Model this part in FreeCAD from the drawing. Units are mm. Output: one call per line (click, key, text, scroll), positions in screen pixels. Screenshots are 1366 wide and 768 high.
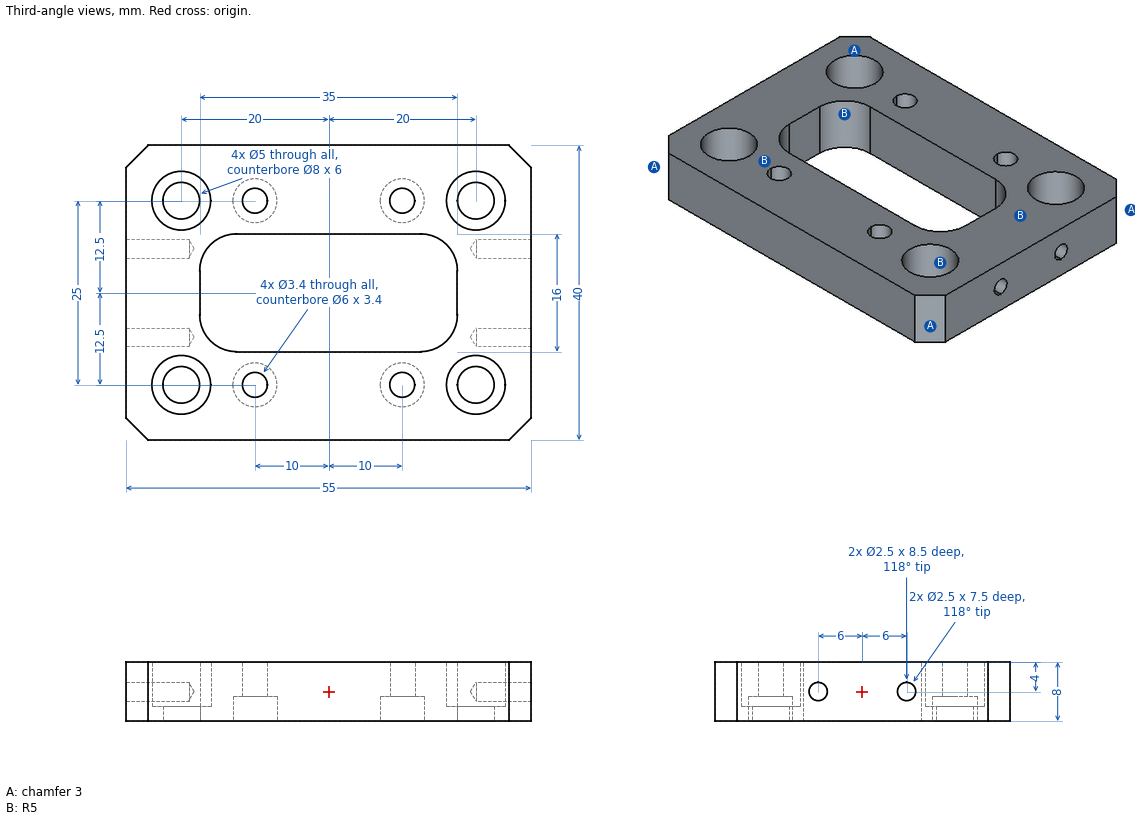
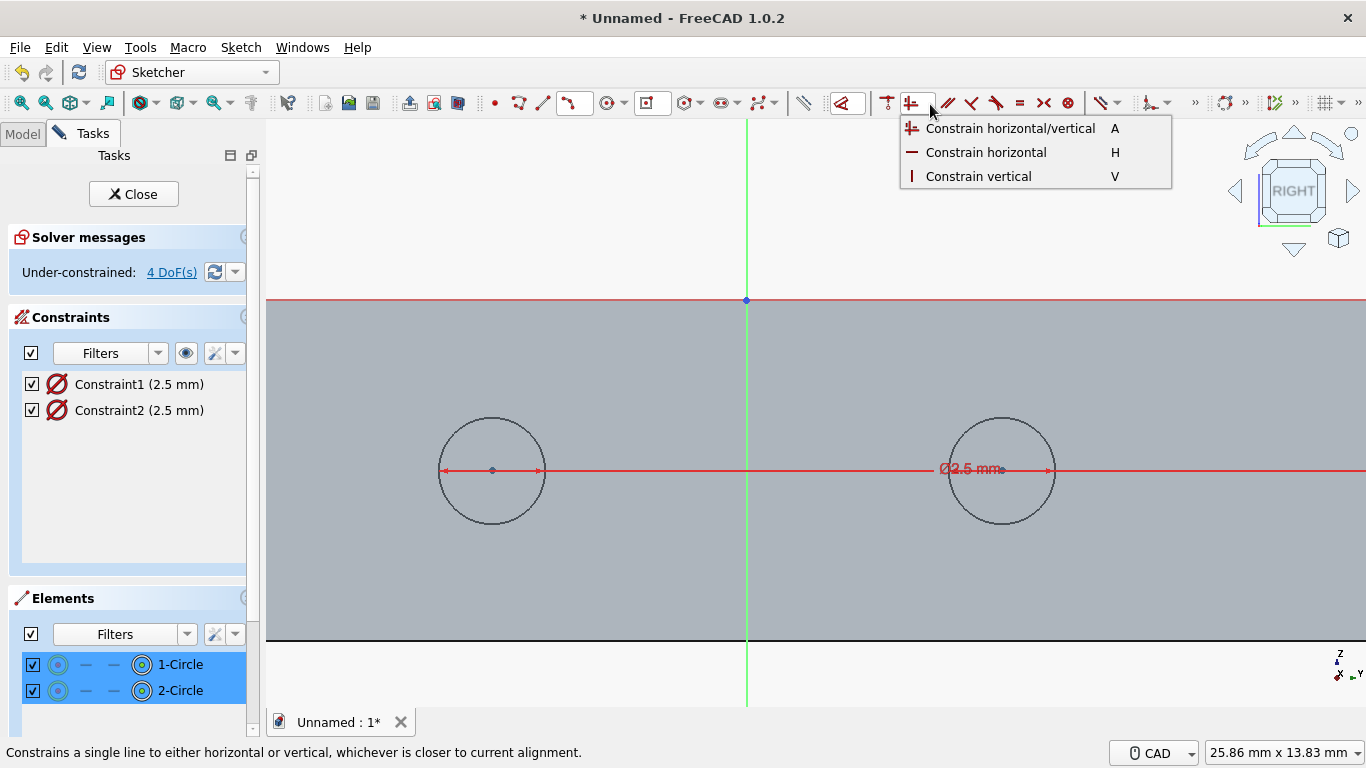
click(1036, 152)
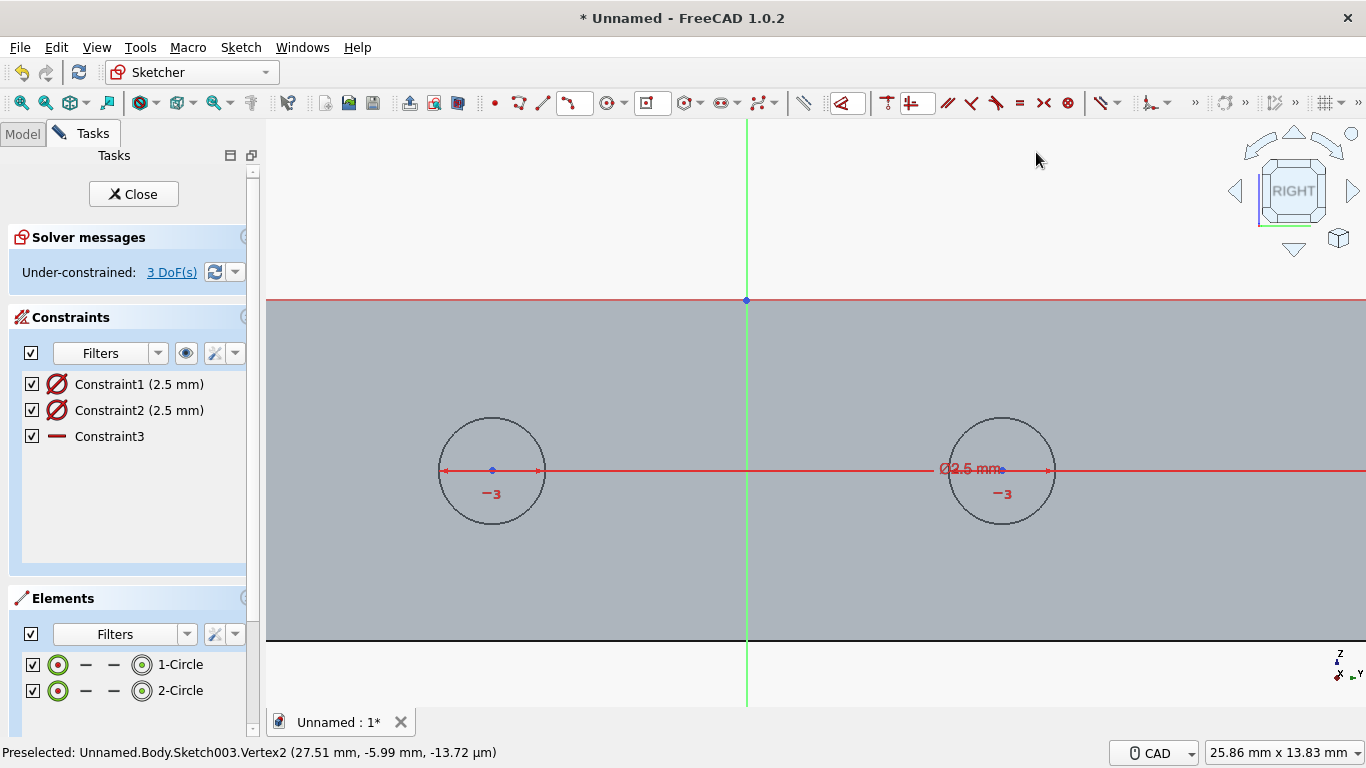
click(1002, 471)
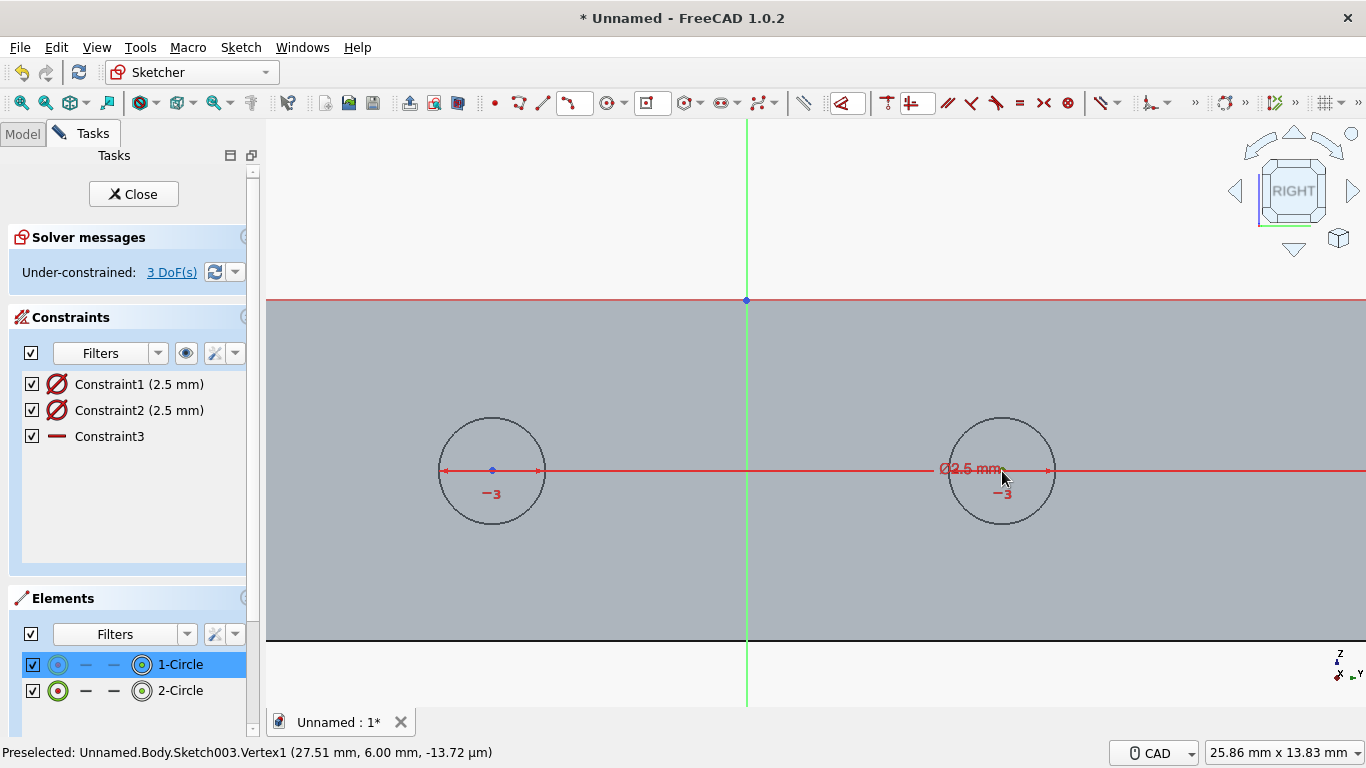
click(860, 104)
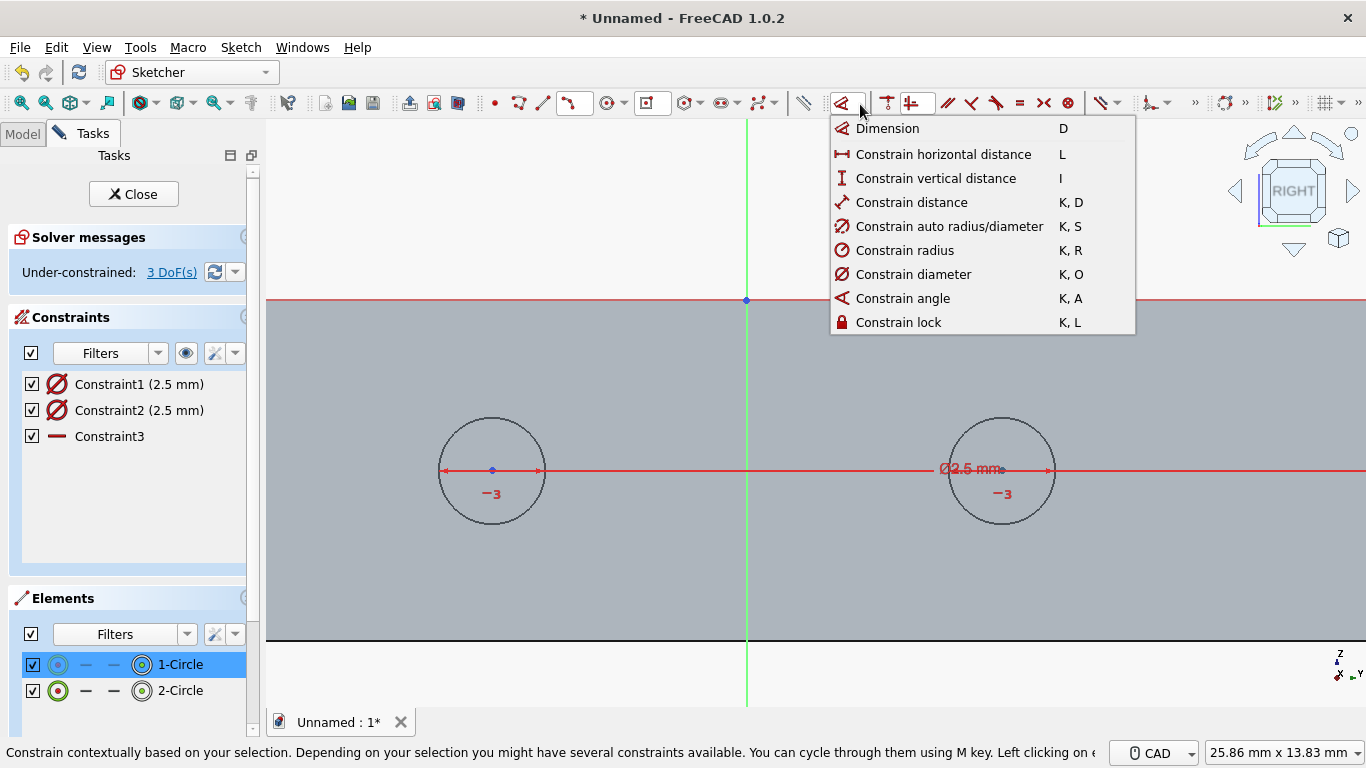
click(983, 154)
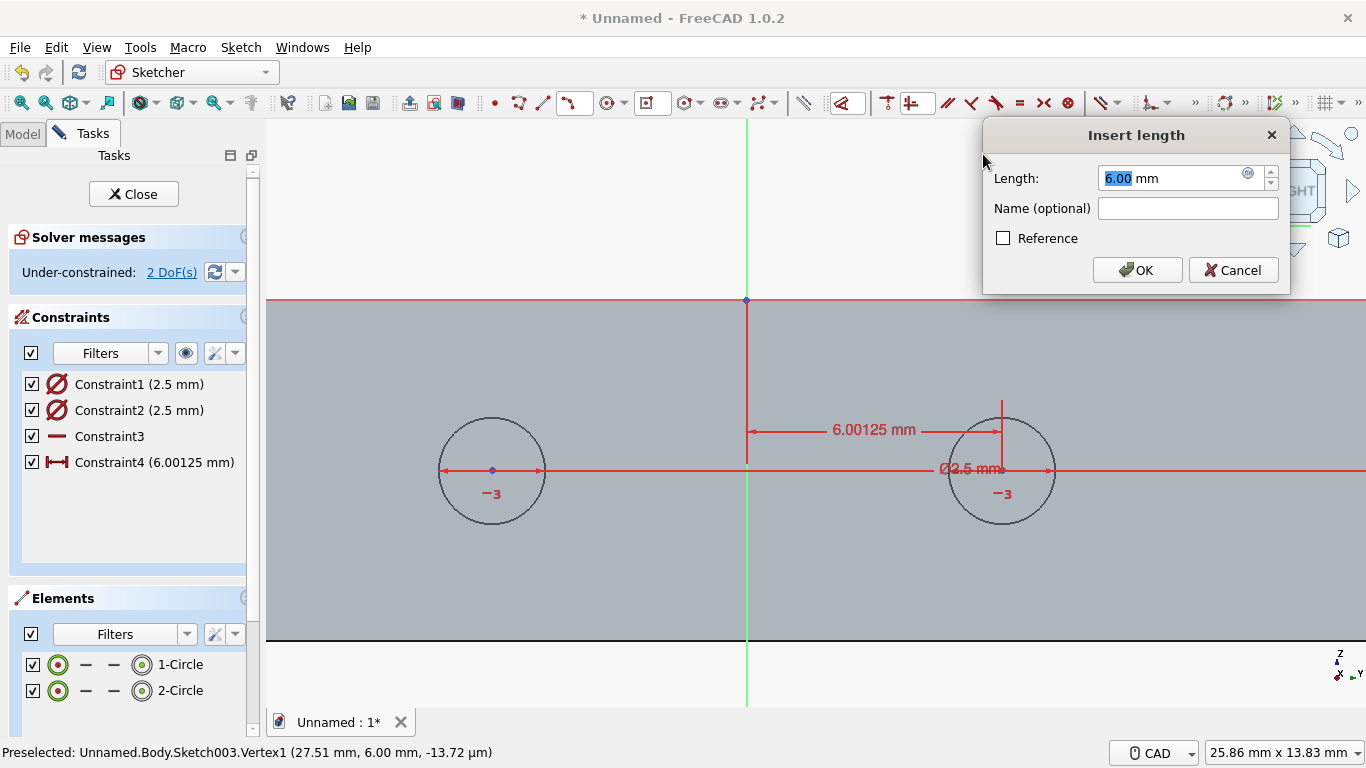
text(6)
key(Return)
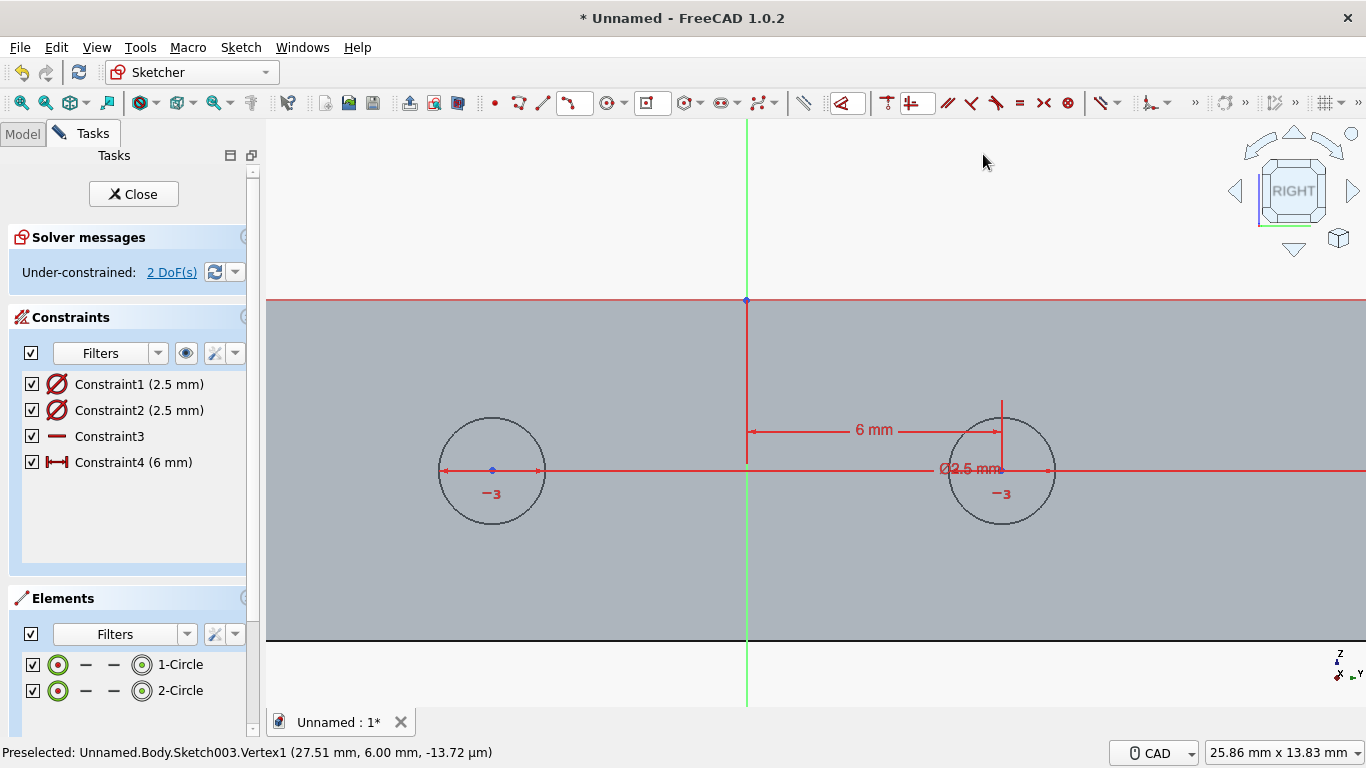
click(1002, 471)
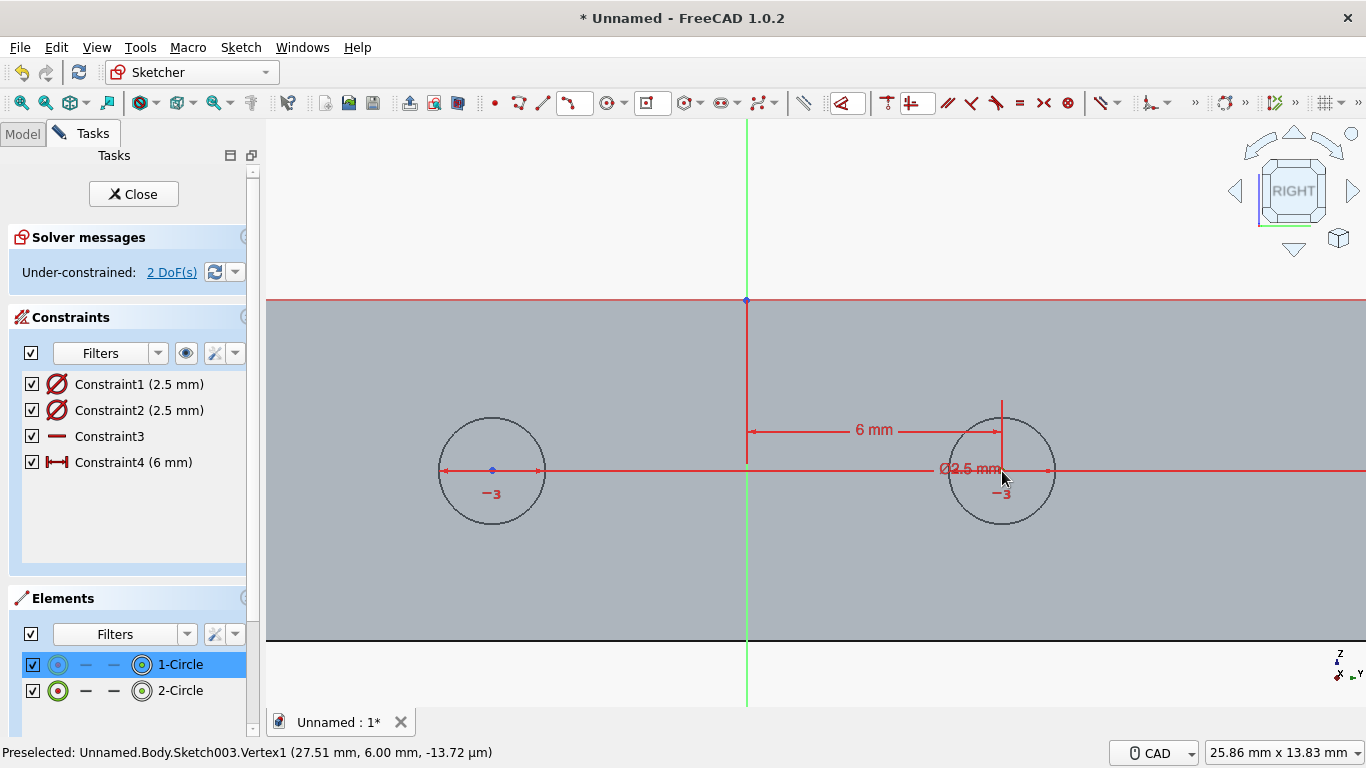
key(i)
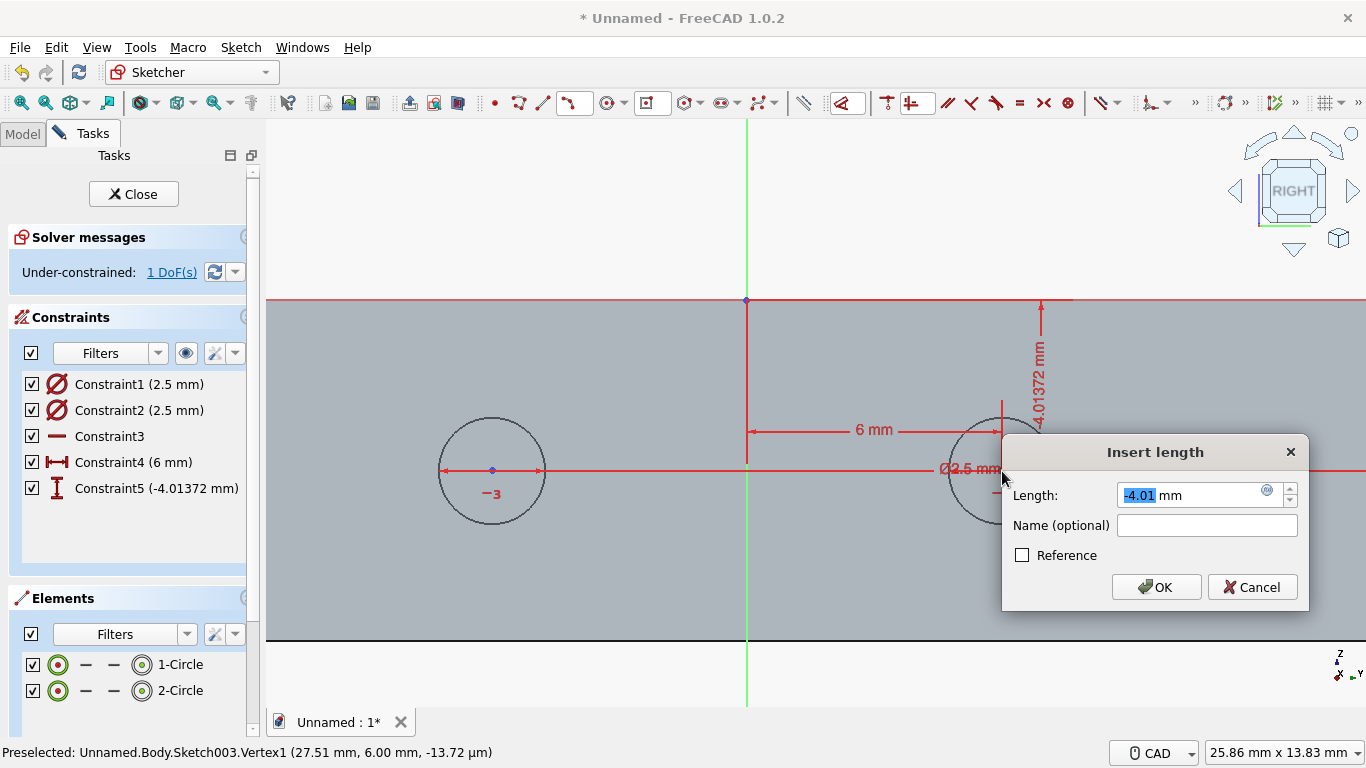
text(-4)
key(Return)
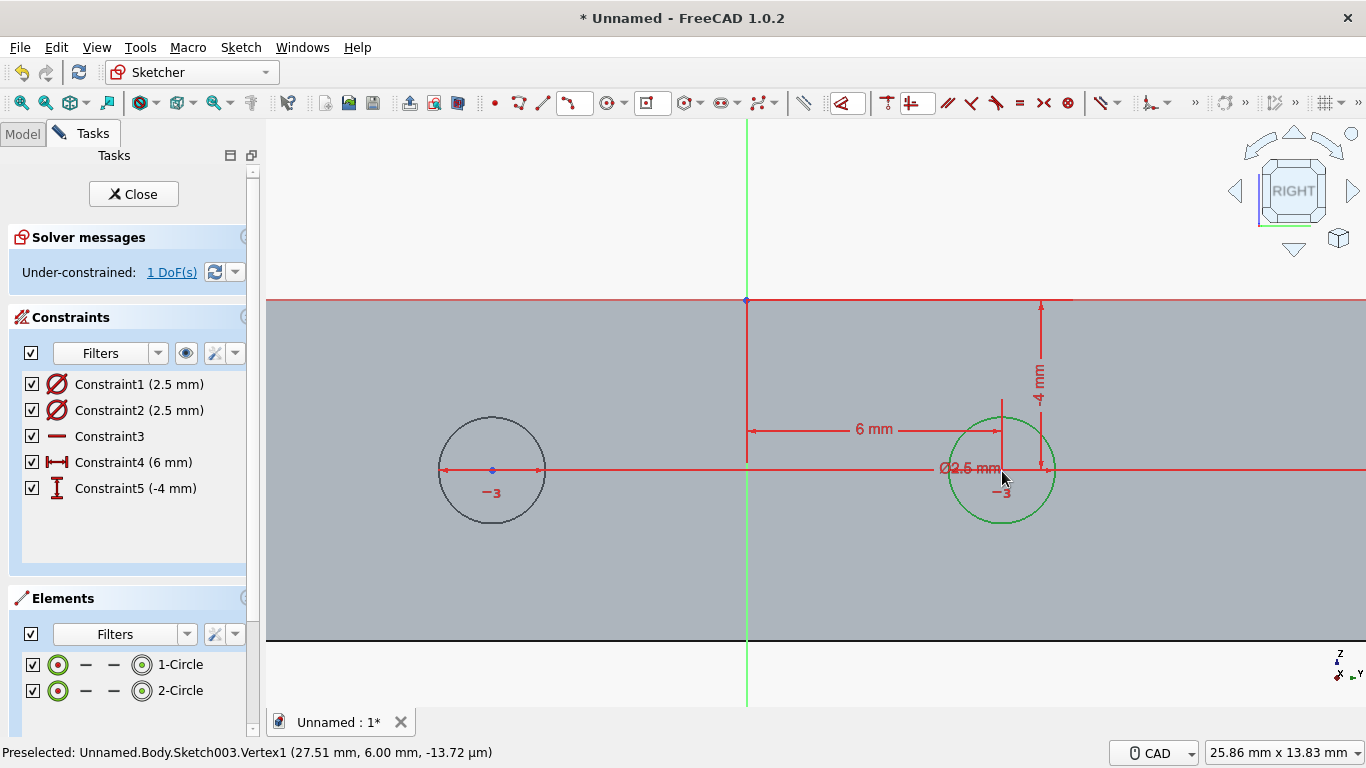
click(492, 470)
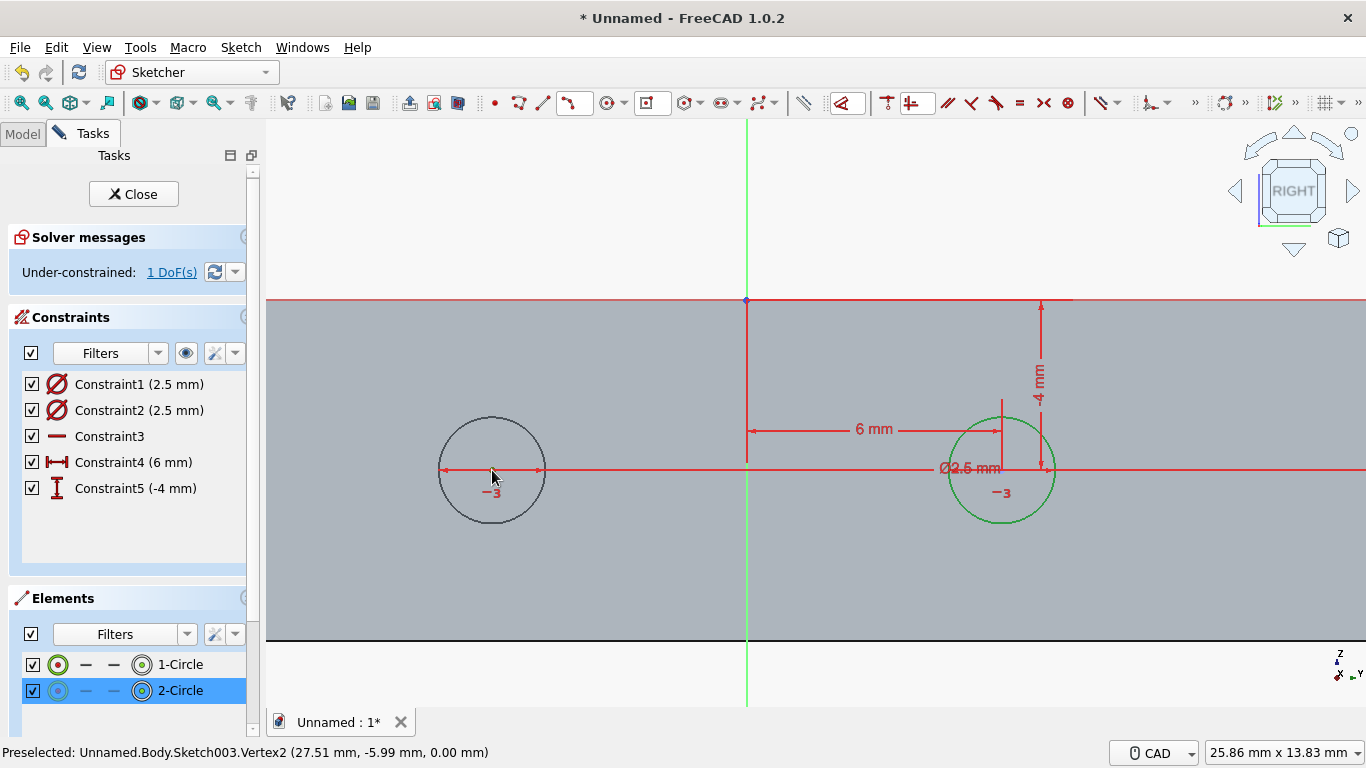
click(860, 104)